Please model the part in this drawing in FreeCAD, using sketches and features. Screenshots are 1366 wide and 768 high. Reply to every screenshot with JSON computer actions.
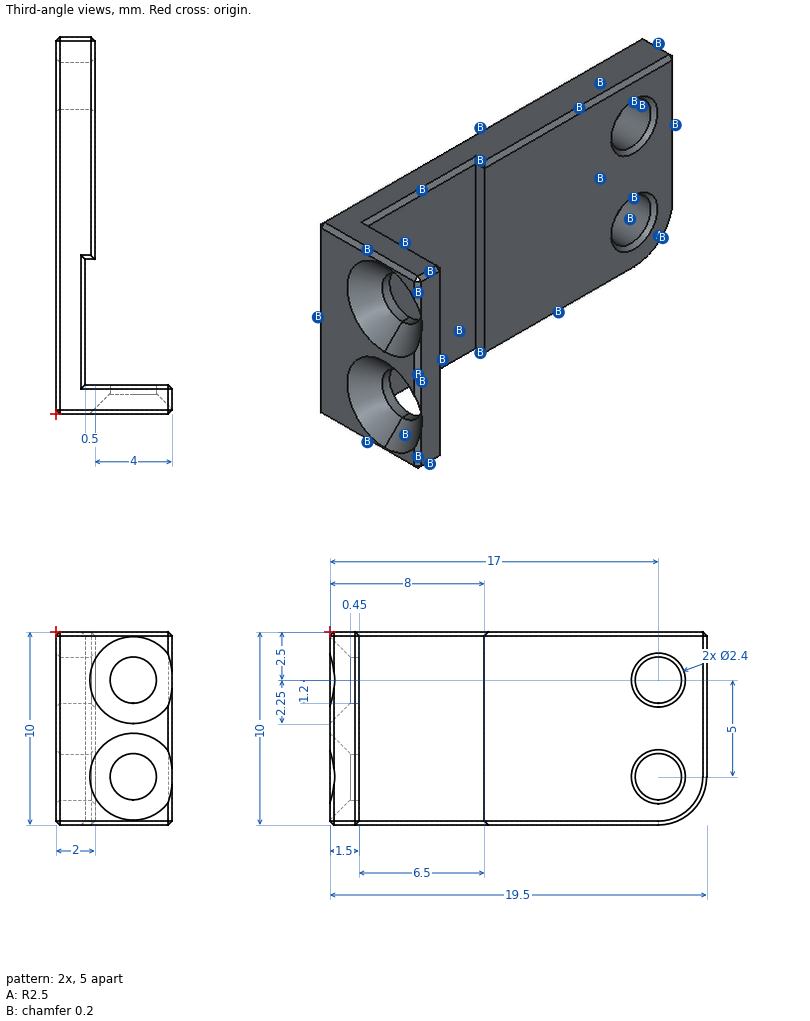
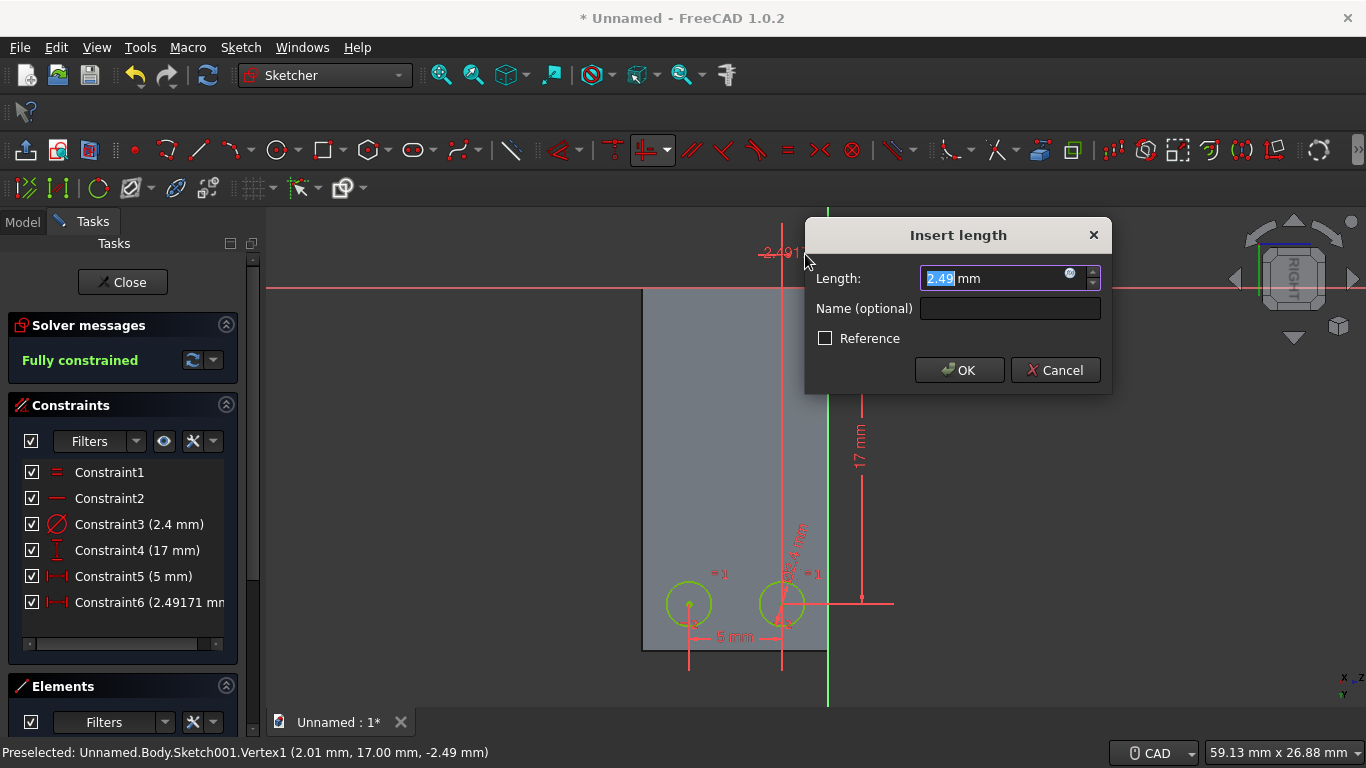
{"action": "type", "text": "2.5"}
{"action": "key", "text": "Return"}
{"action": "key", "text": "Escape"}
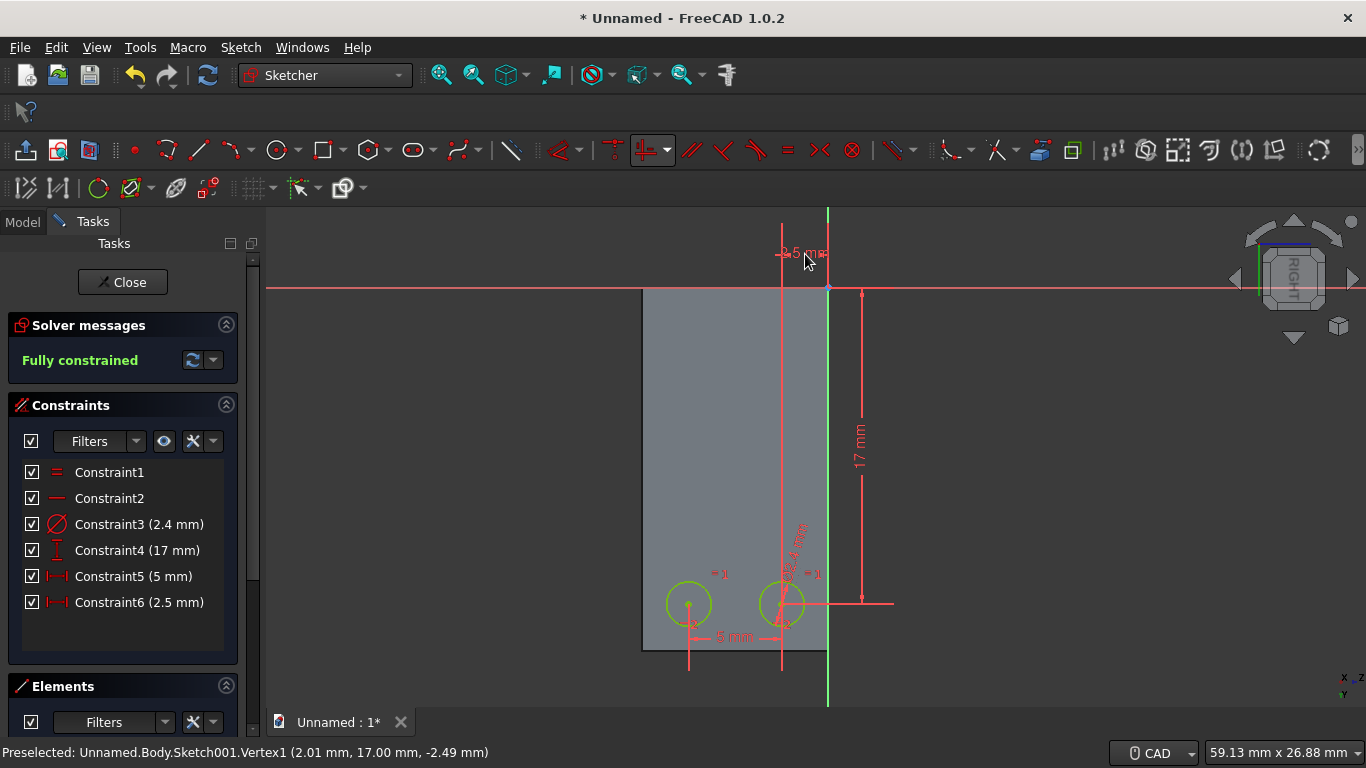
{"action": "left_click", "coordinate": [123, 282]}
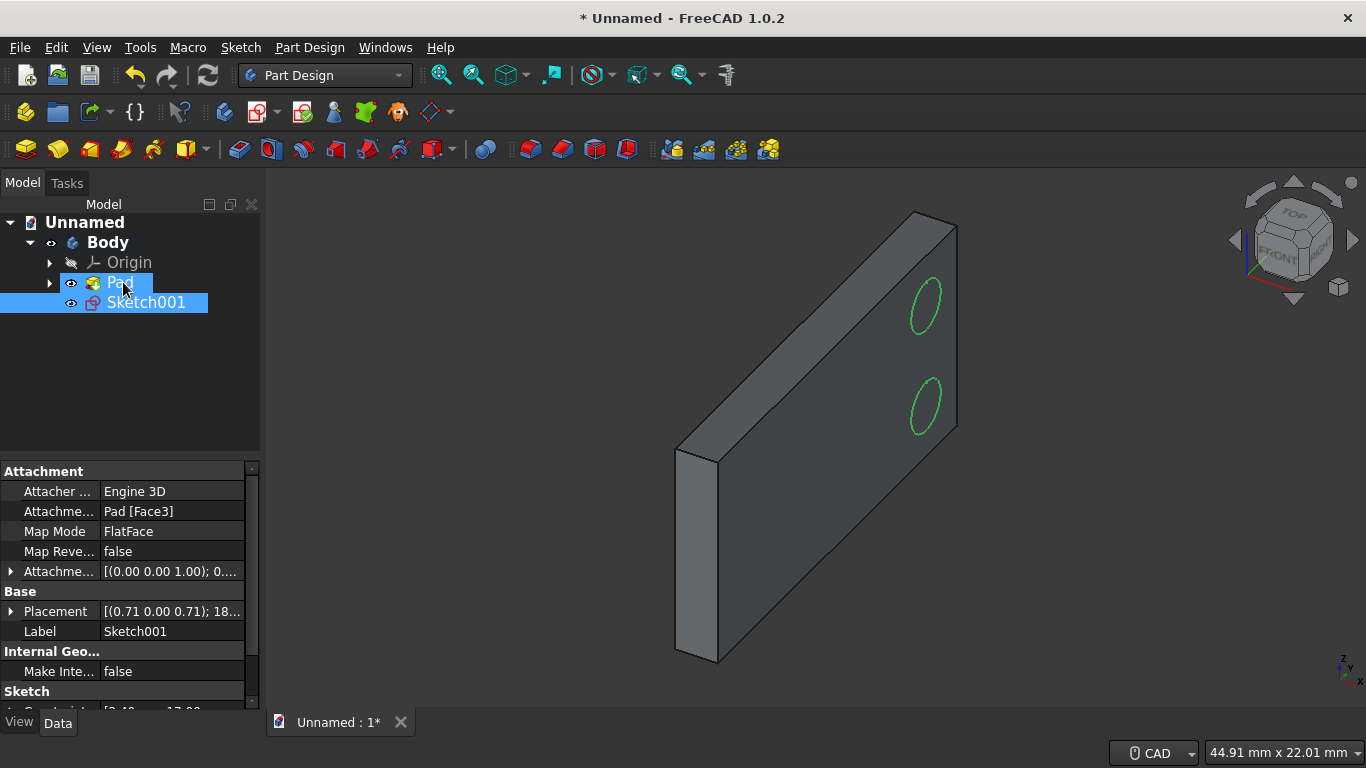
{"action": "left_click", "coordinate": [240, 150]}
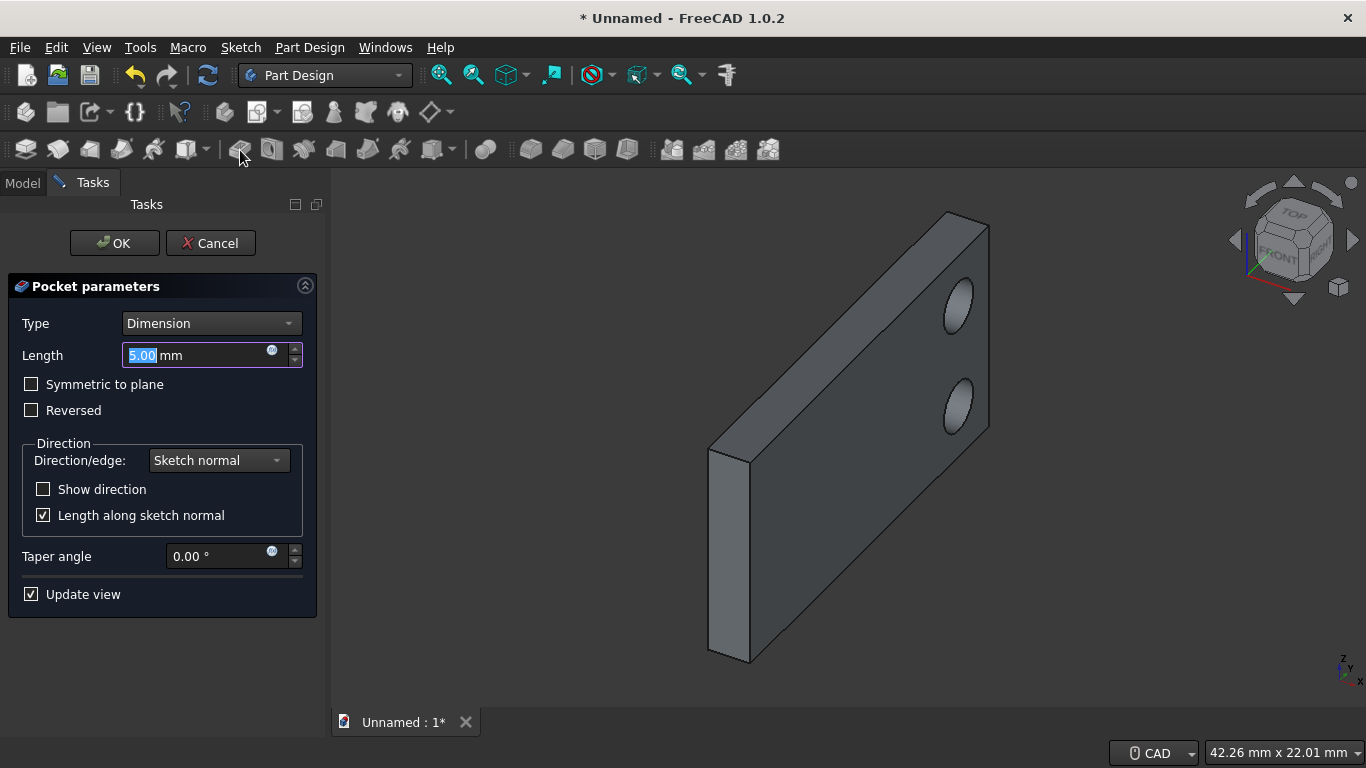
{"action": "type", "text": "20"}
{"action": "key", "text": "Tab"}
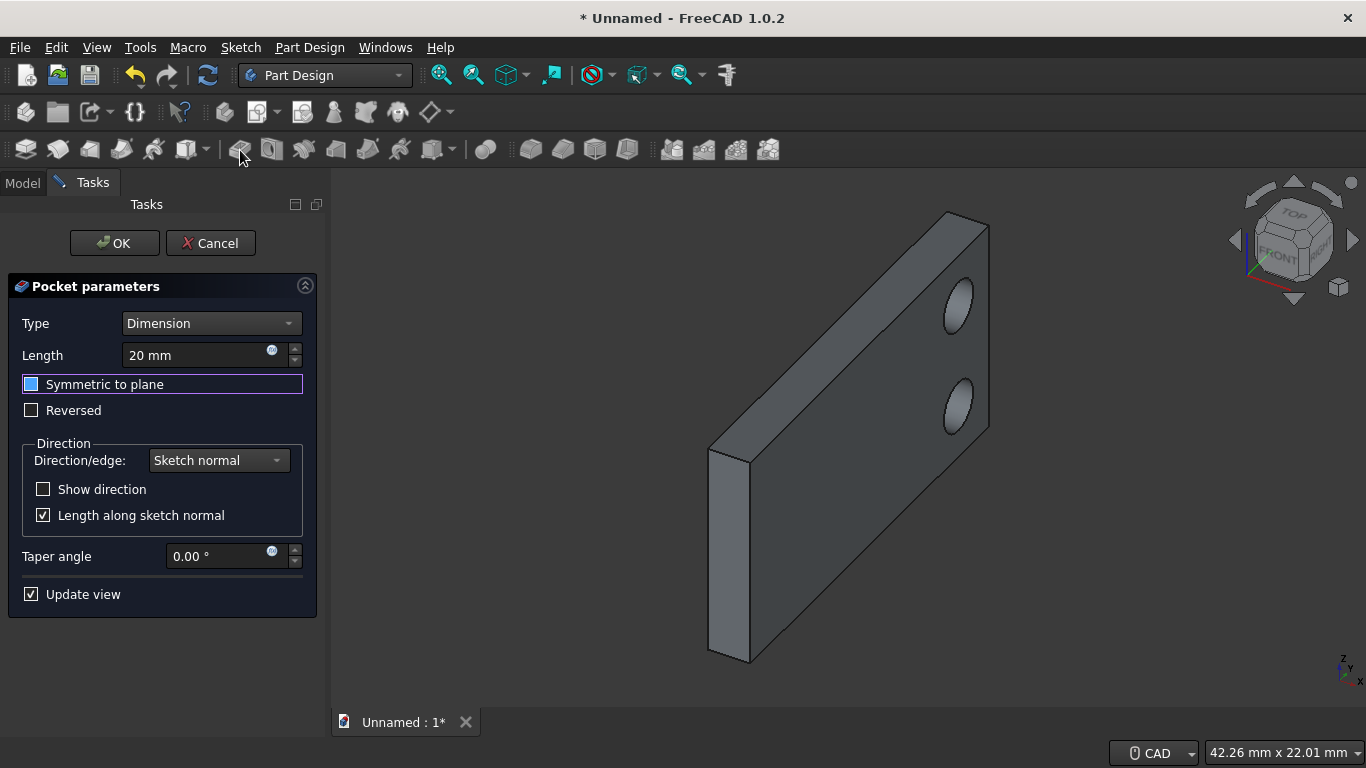
{"action": "left_click", "coordinate": [115, 243]}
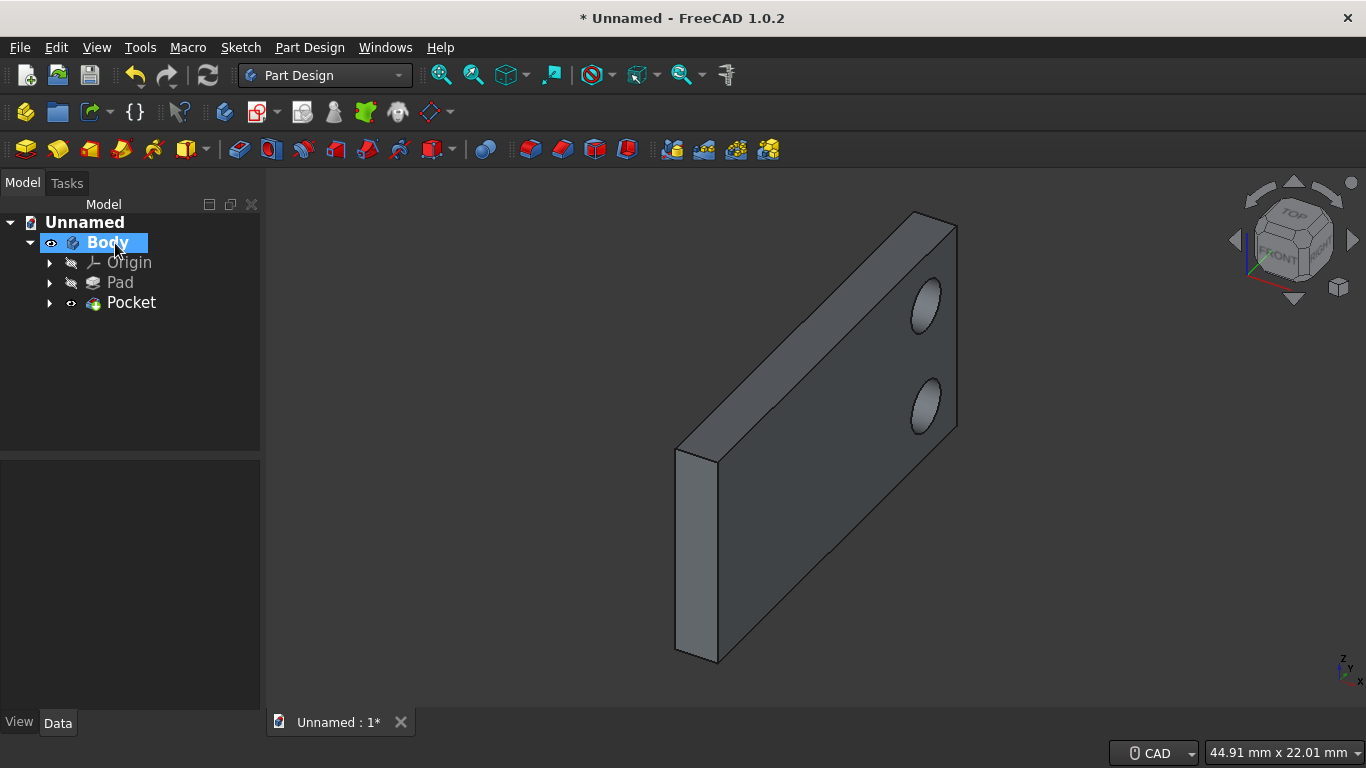
{"action": "left_click", "coordinate": [803, 477]}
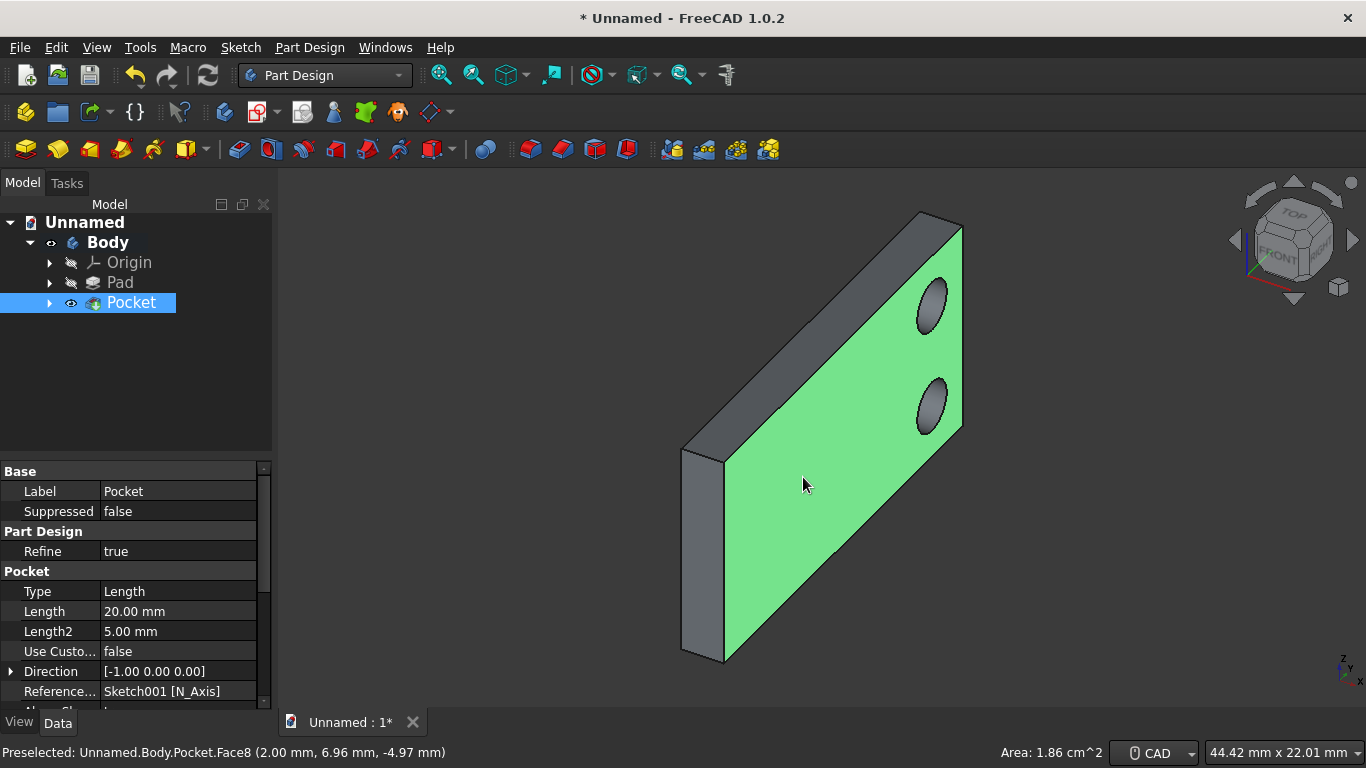
{"action": "left_click", "coordinate": [258, 112]}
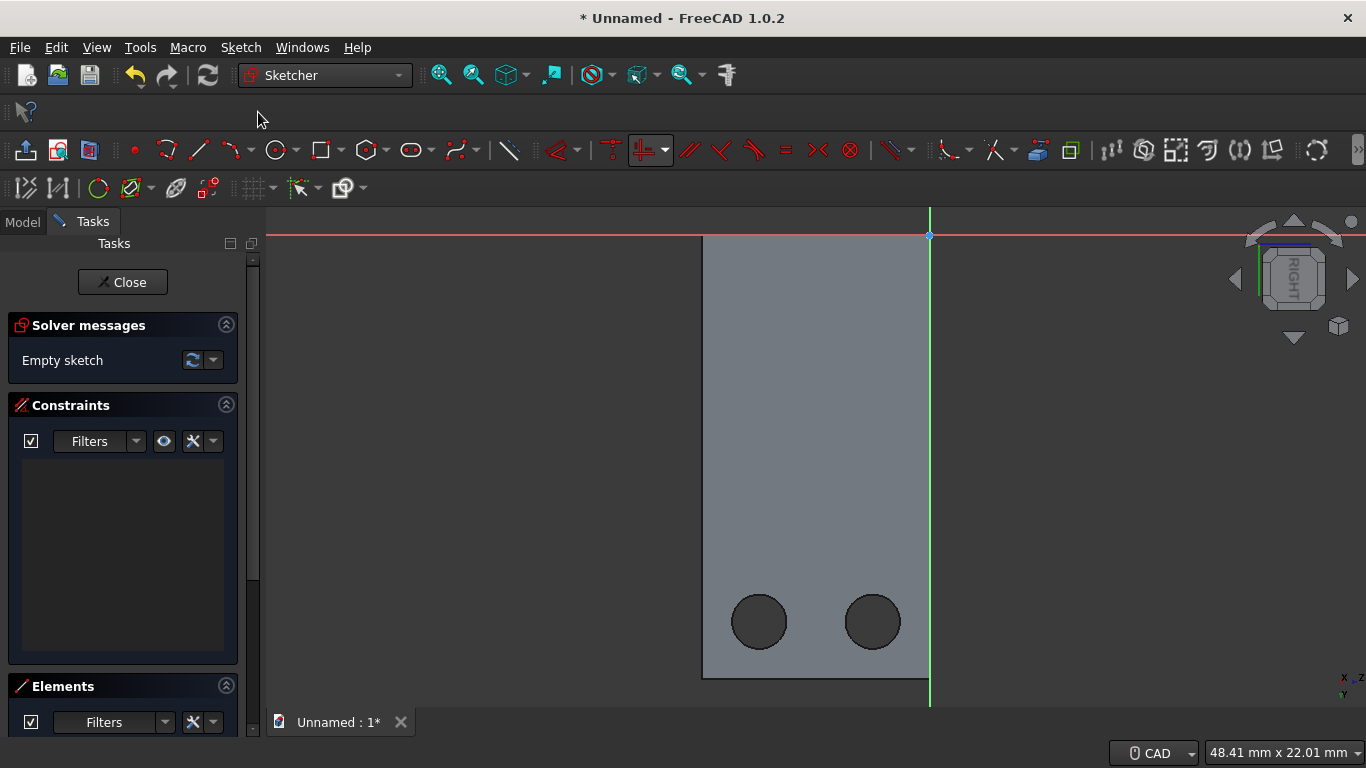
{"action": "scroll", "coordinate": [748, 457], "scroll_direction": "down", "scroll_amount": 5}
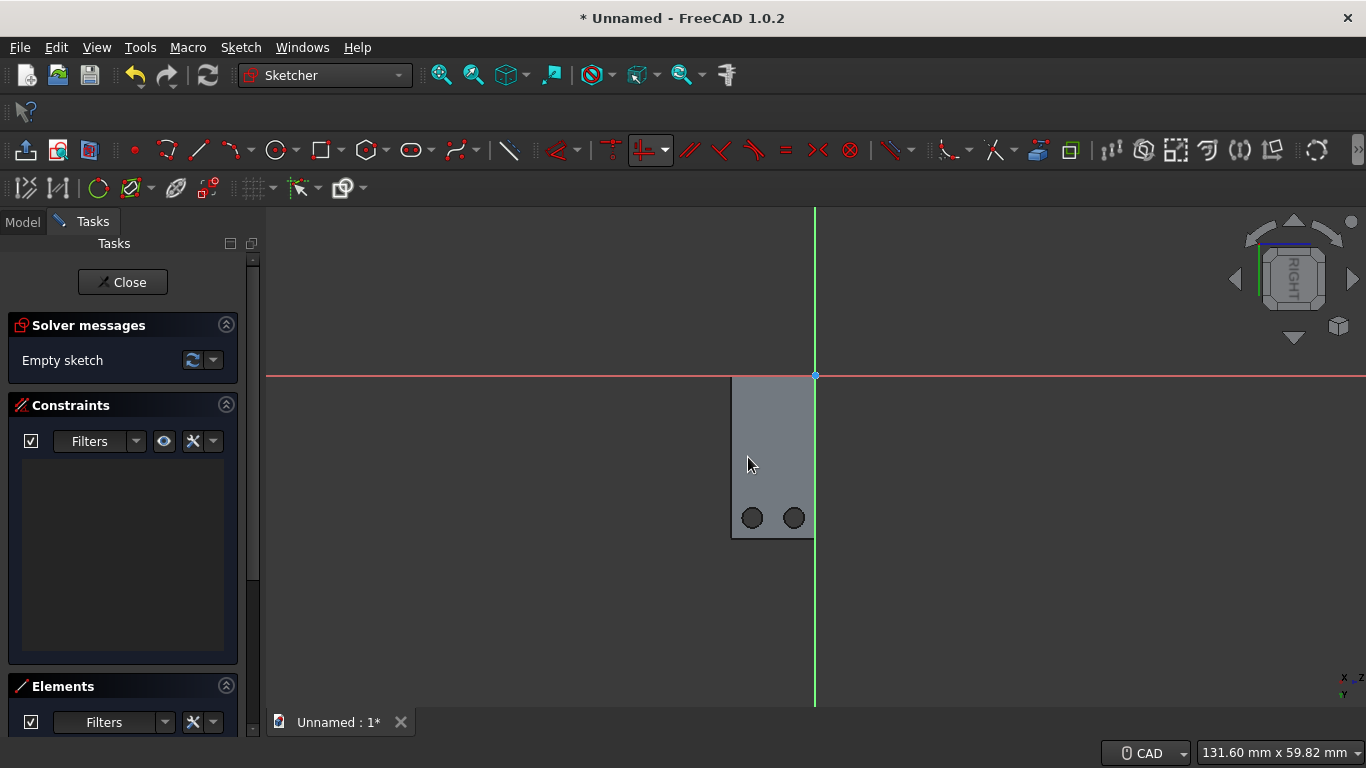
{"action": "scroll", "coordinate": [777, 370], "scroll_direction": "up", "scroll_amount": 10}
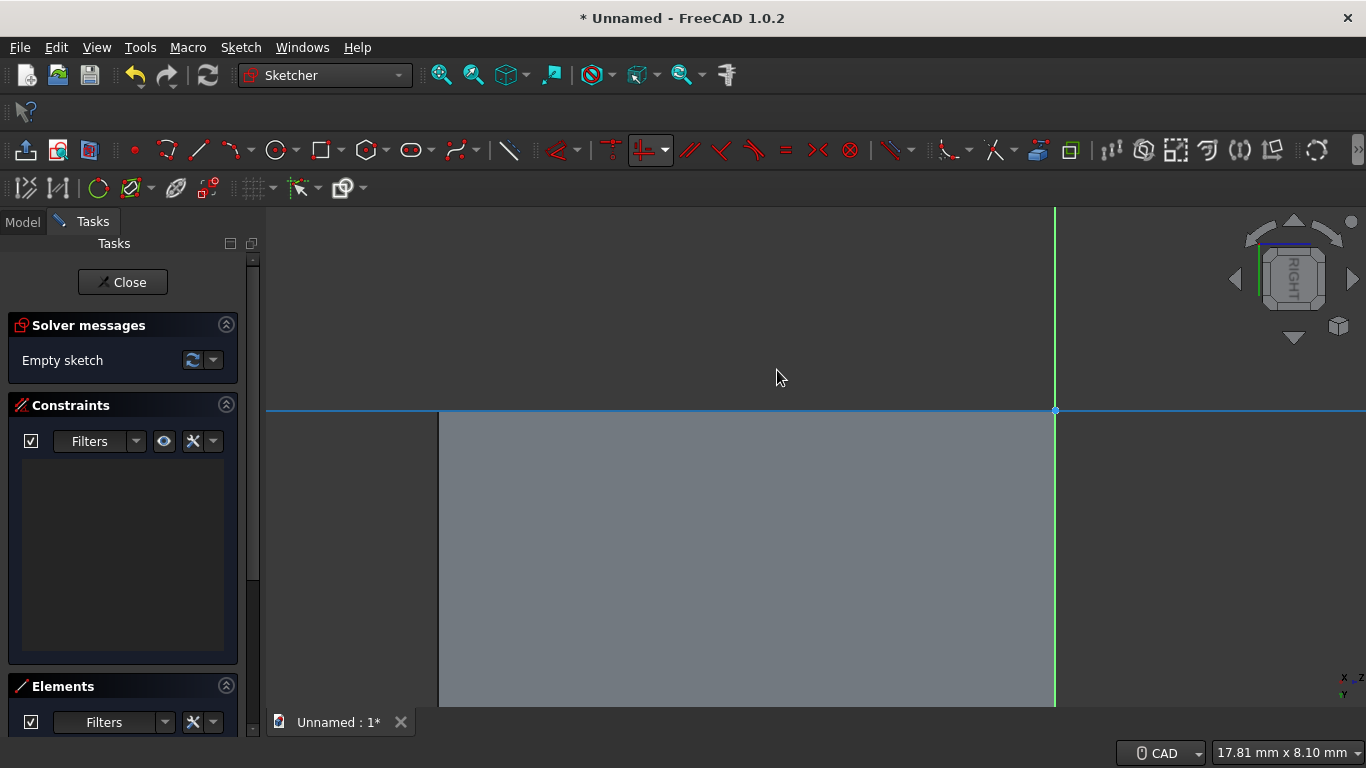
{"action": "left_click", "coordinate": [322, 150]}